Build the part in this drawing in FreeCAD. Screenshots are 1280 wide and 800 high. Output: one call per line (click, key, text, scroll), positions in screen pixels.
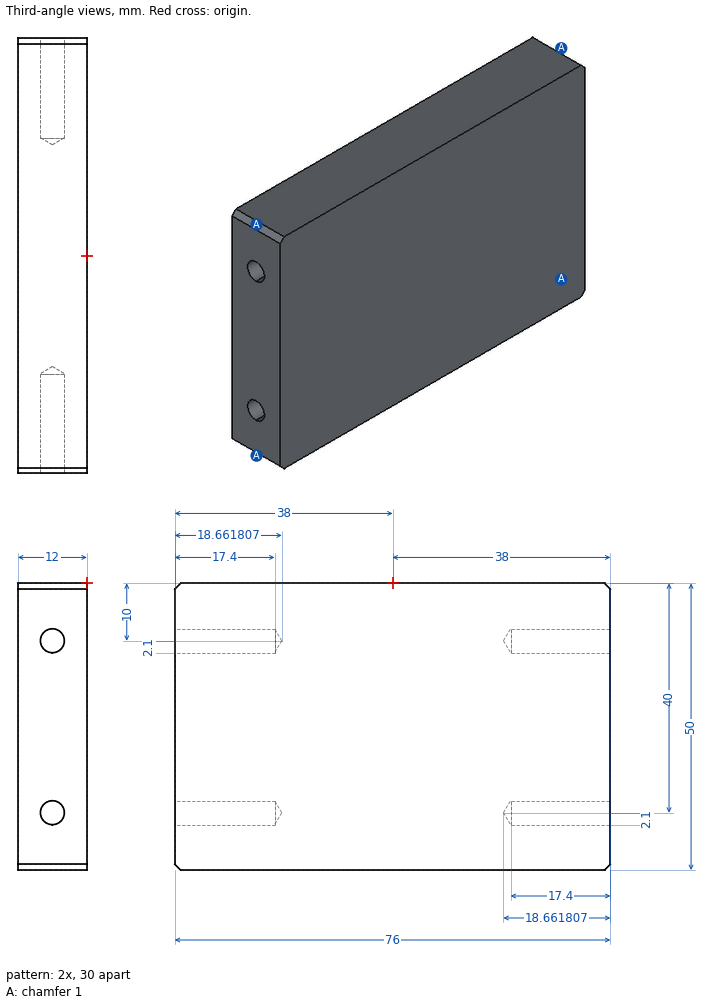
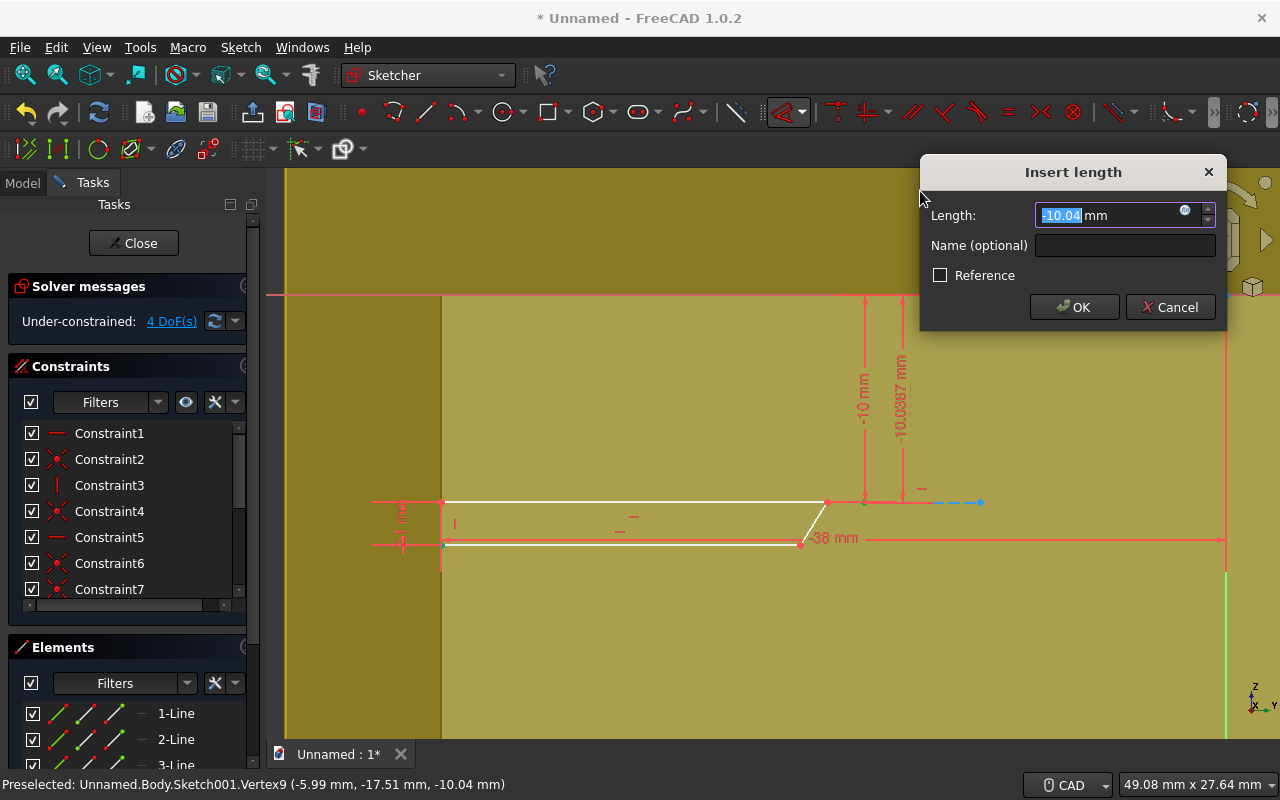
text(-10)
key(Return)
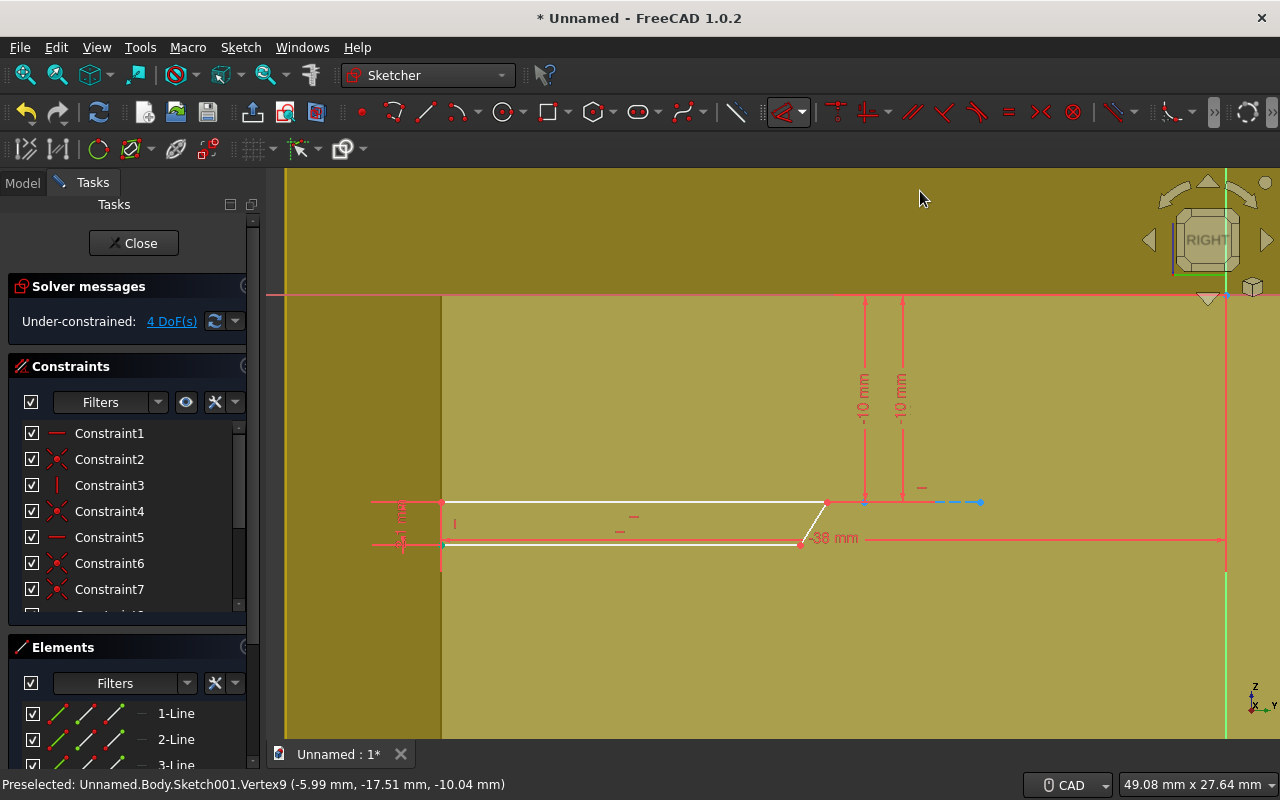
click(549, 545)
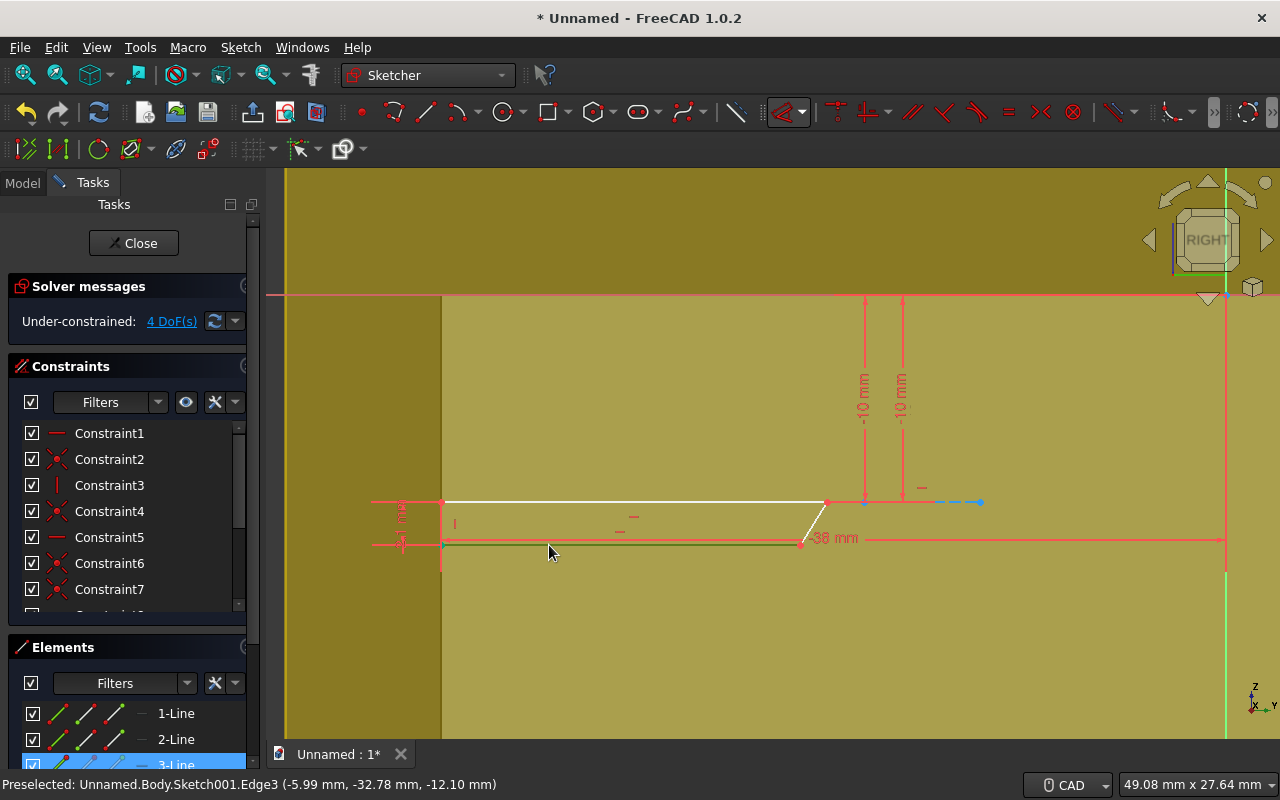
key(l)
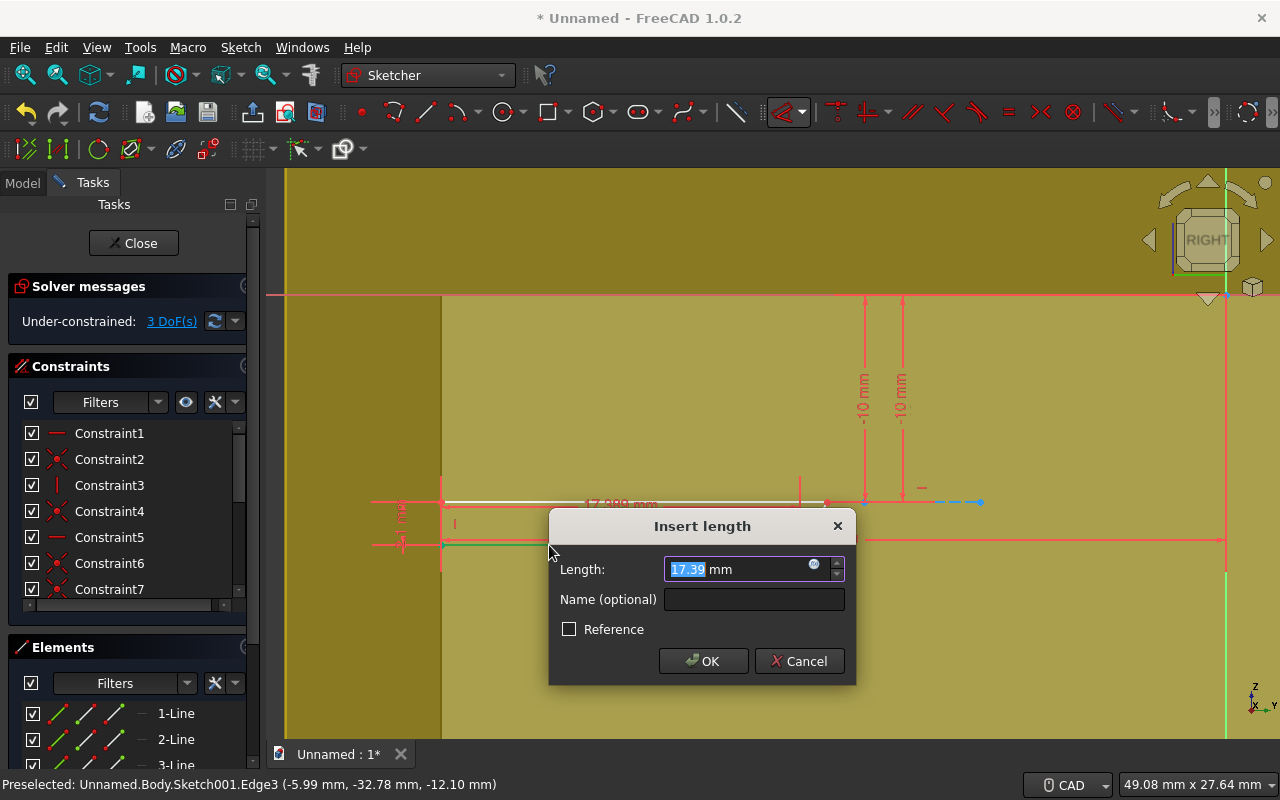
text(17.4)
key(Return)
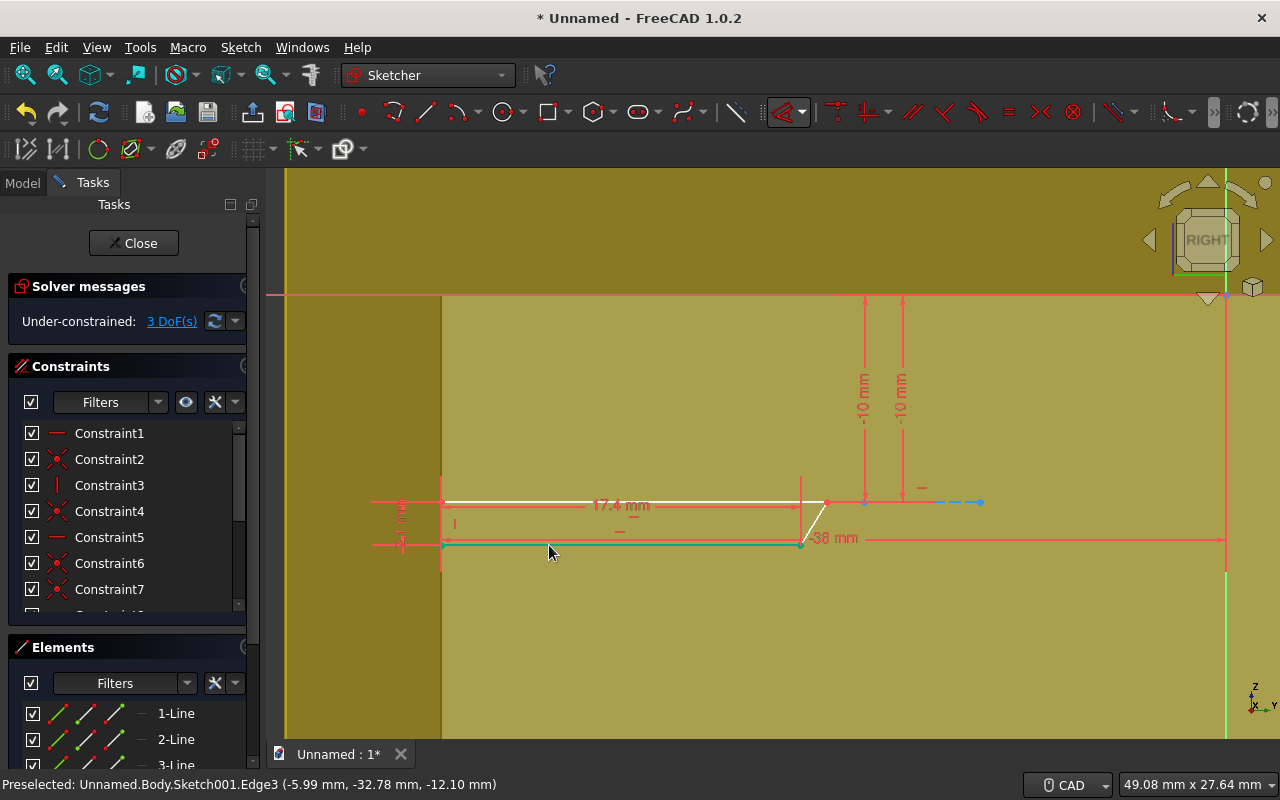
click(711, 502)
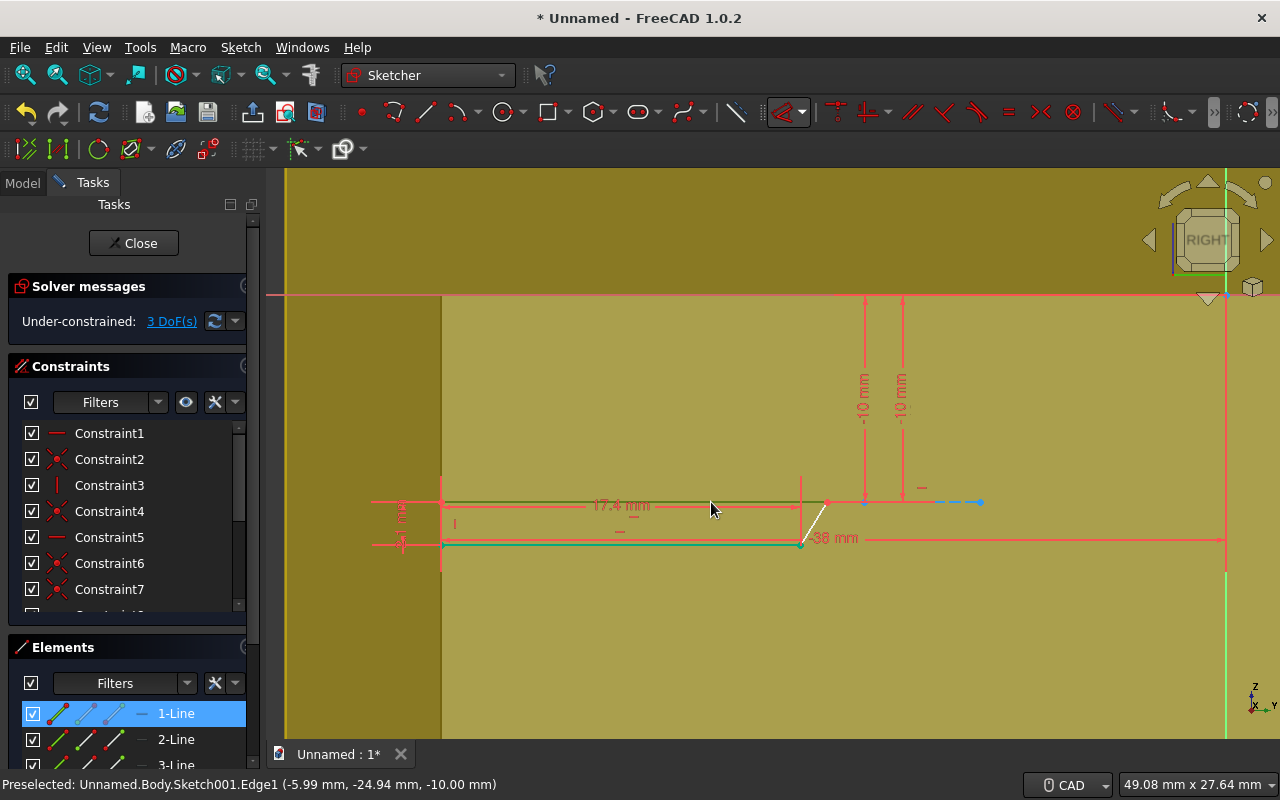
key(l)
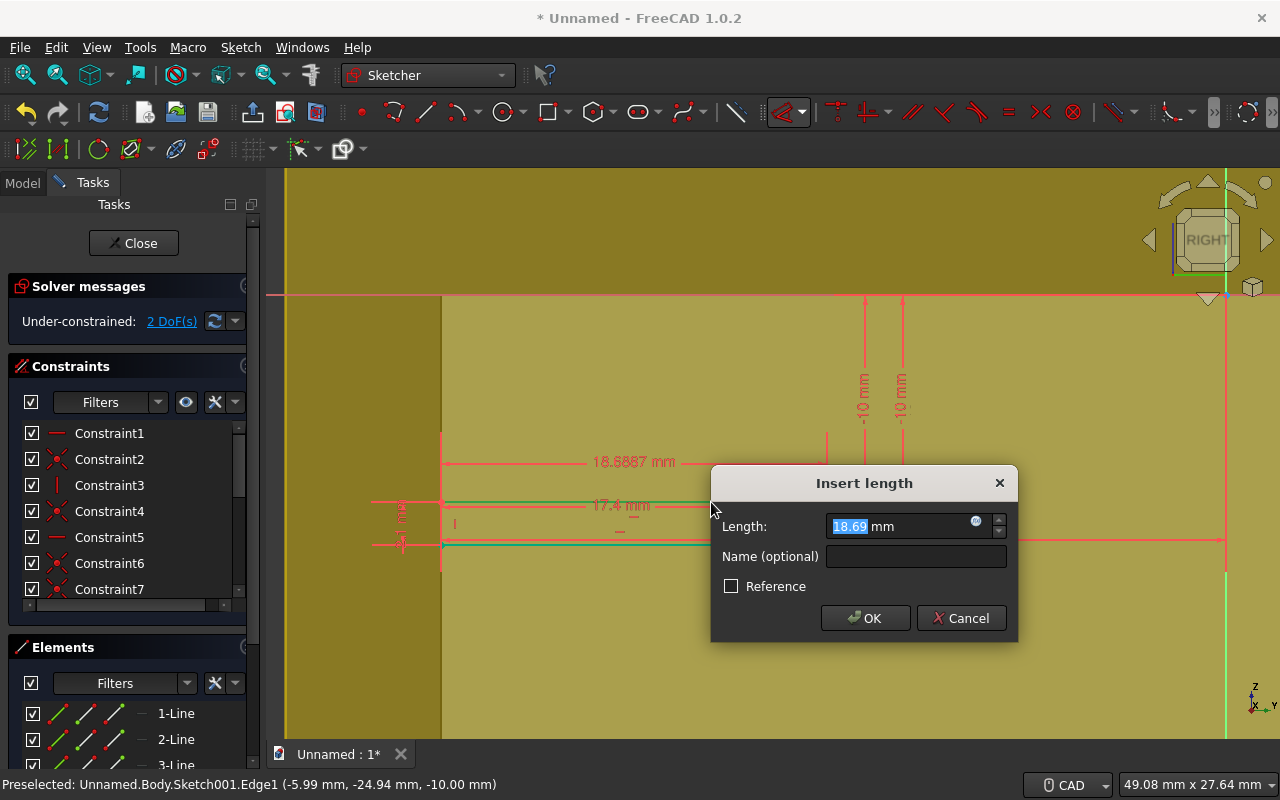
text(18.661807)
key(Return)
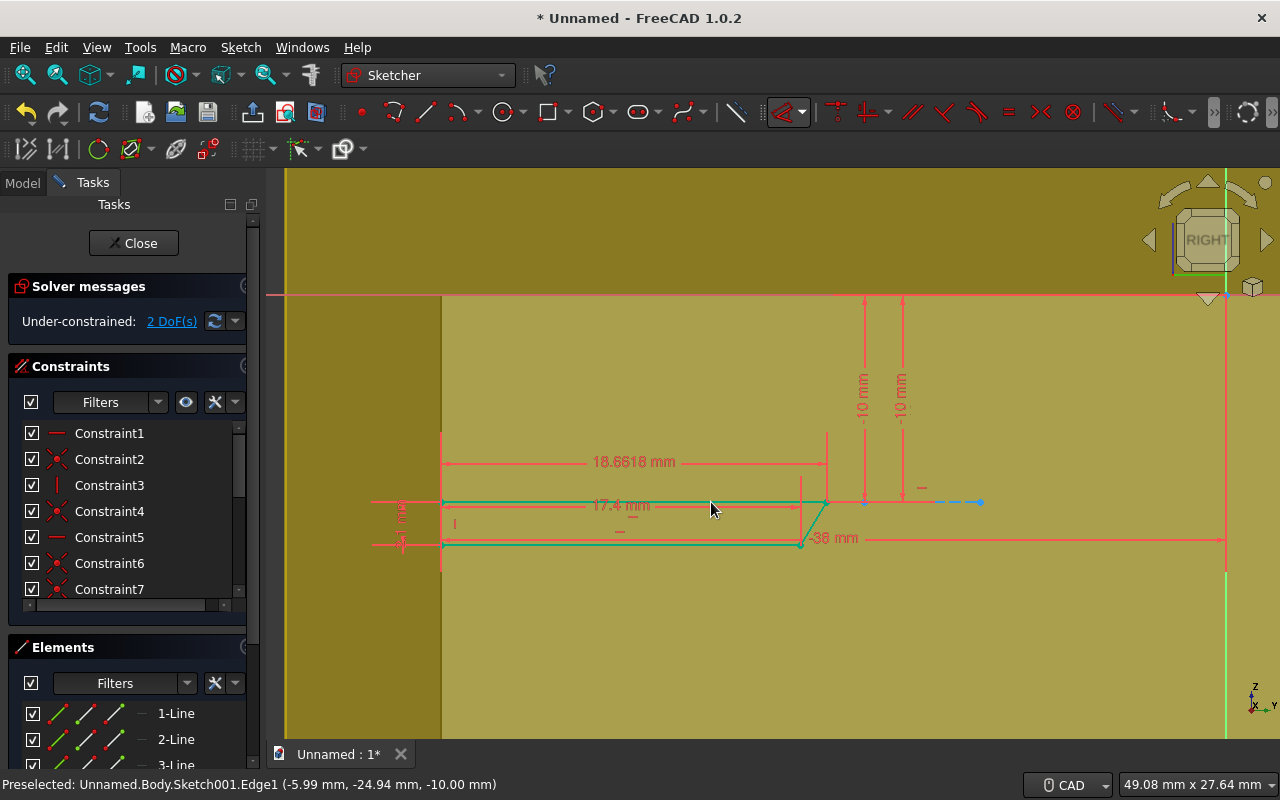
click(134, 243)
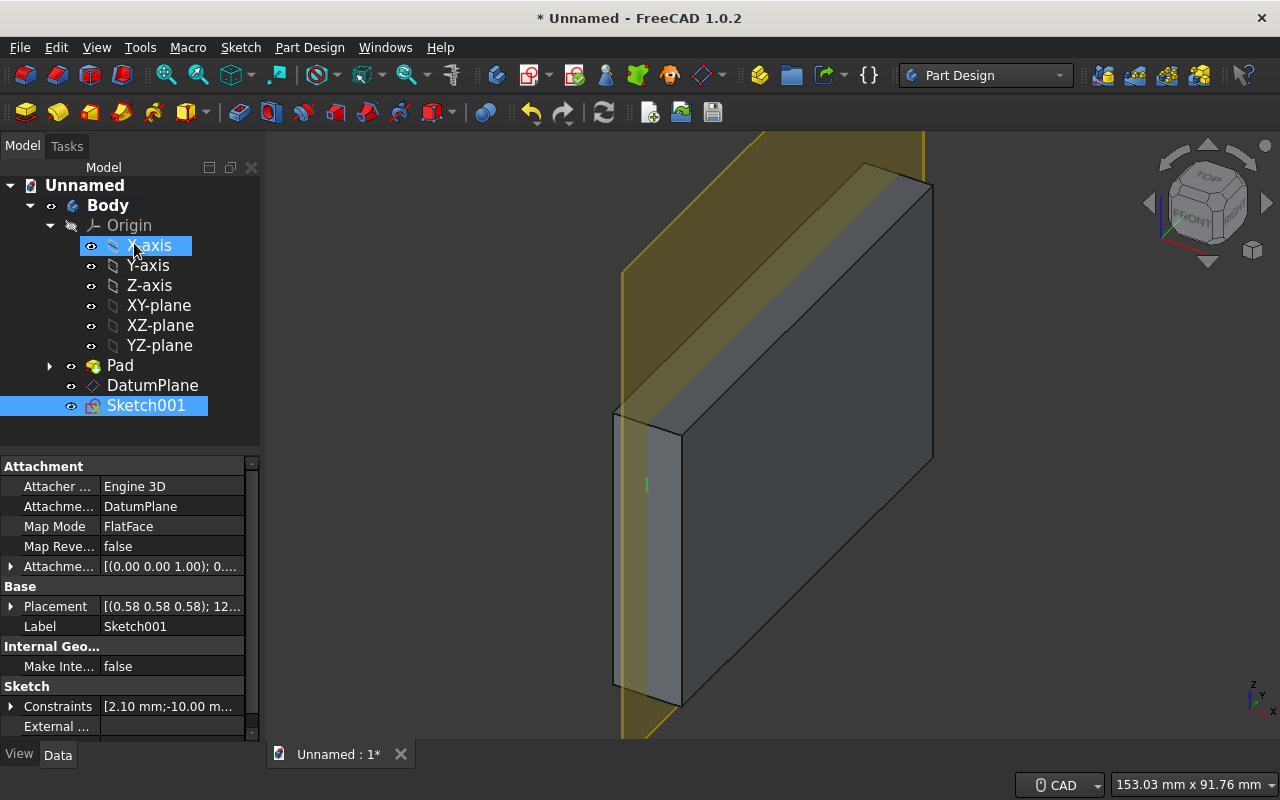
click(304, 112)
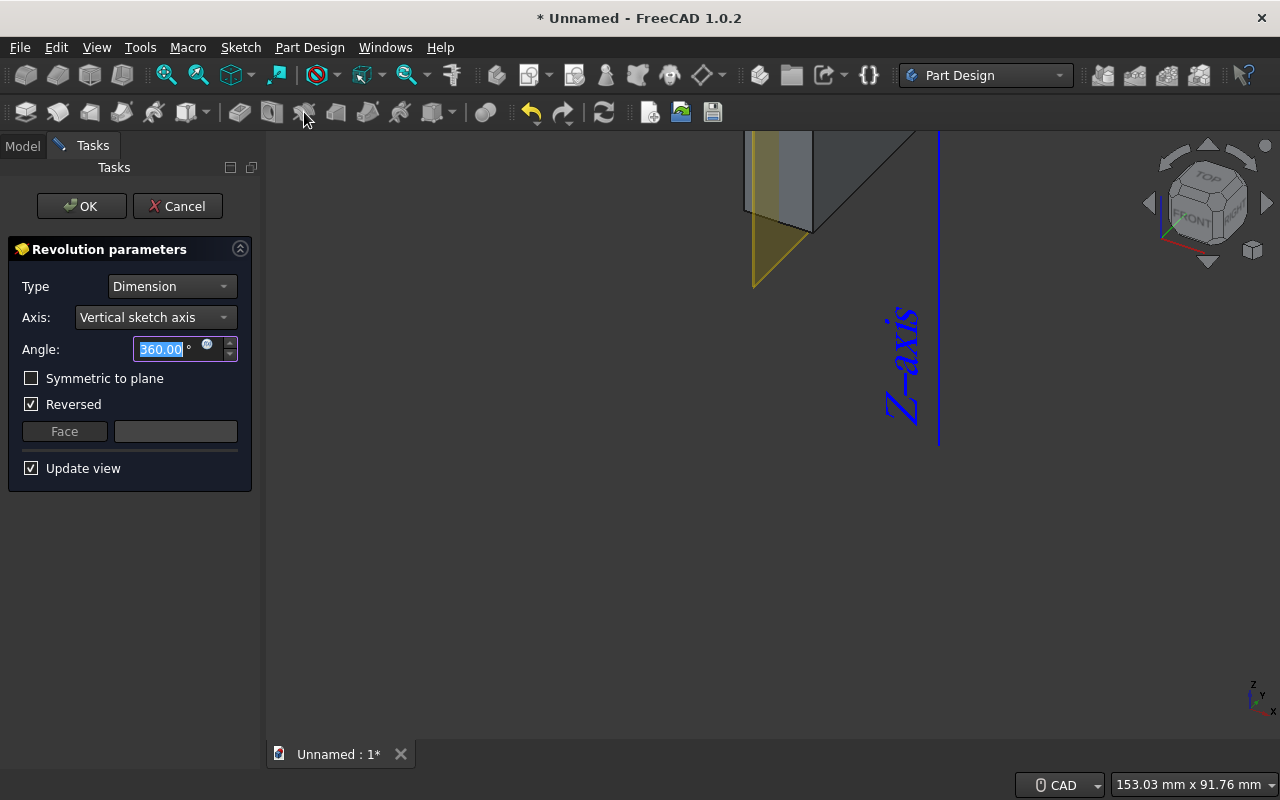
click(156, 318)